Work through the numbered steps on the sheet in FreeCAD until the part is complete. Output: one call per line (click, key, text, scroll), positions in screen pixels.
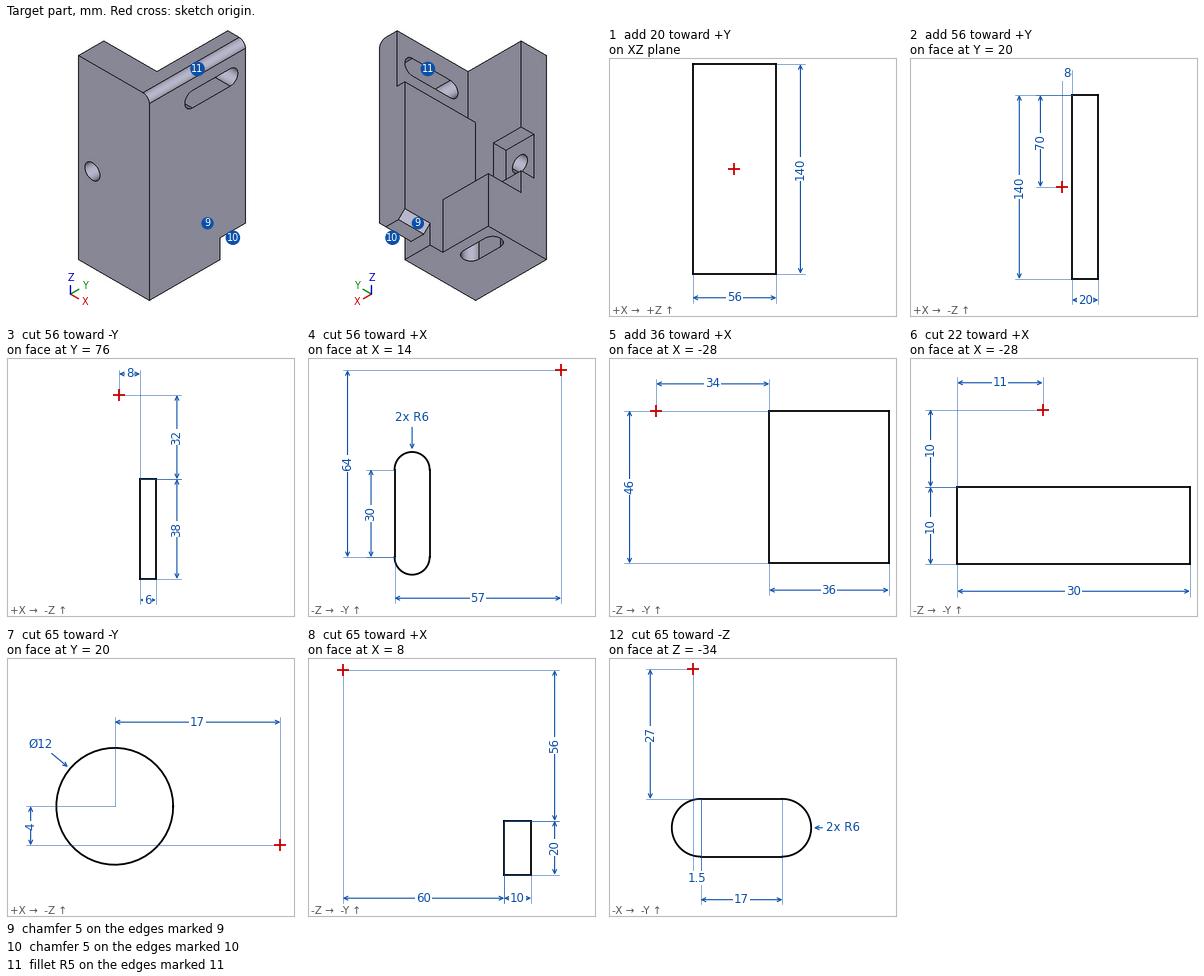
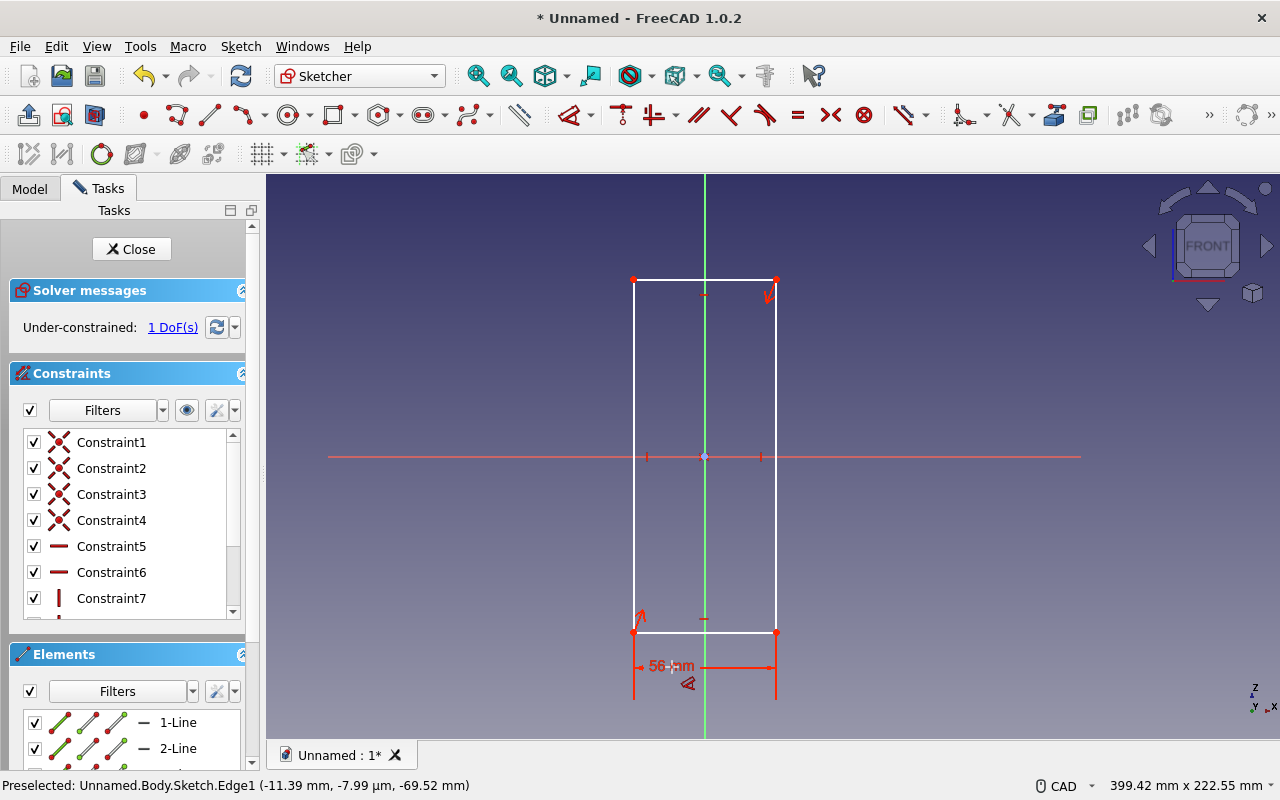
click(776, 527)
click(810, 375)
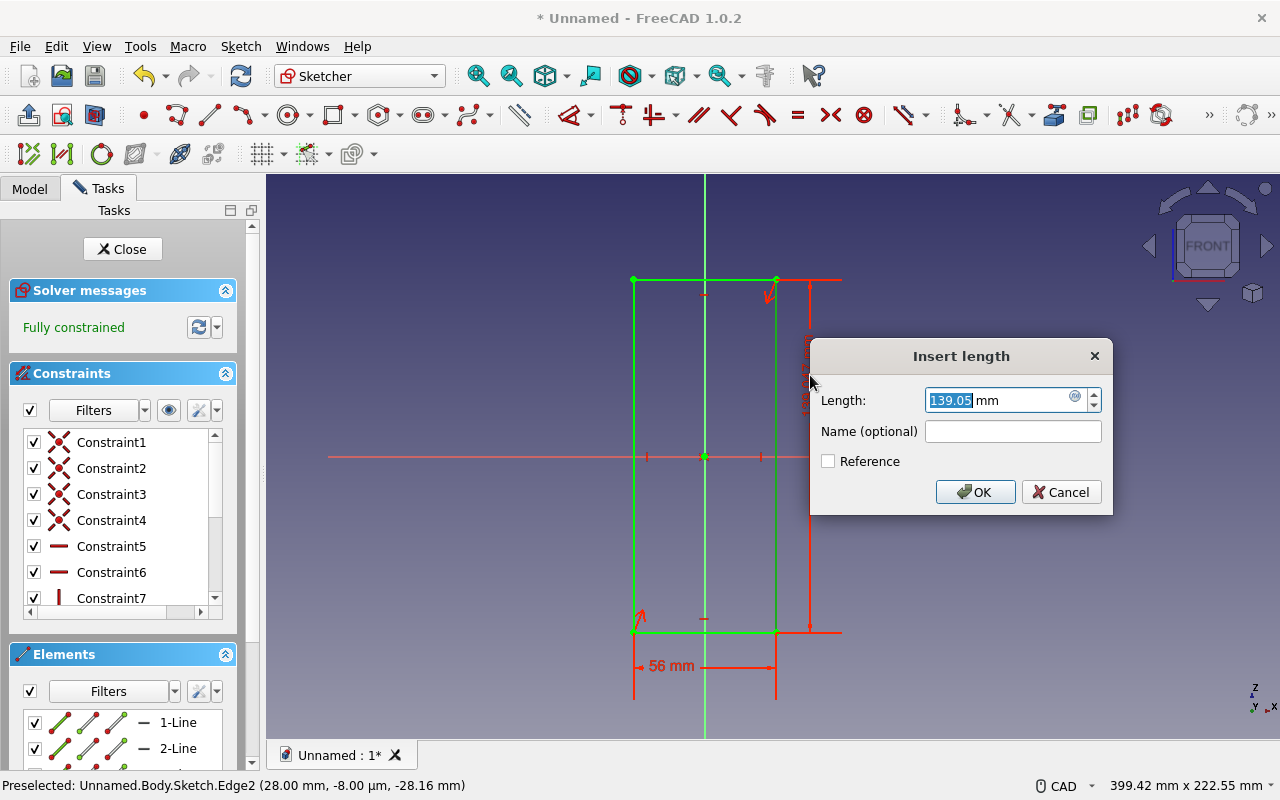
text(140)
key(Return)
key(Escape)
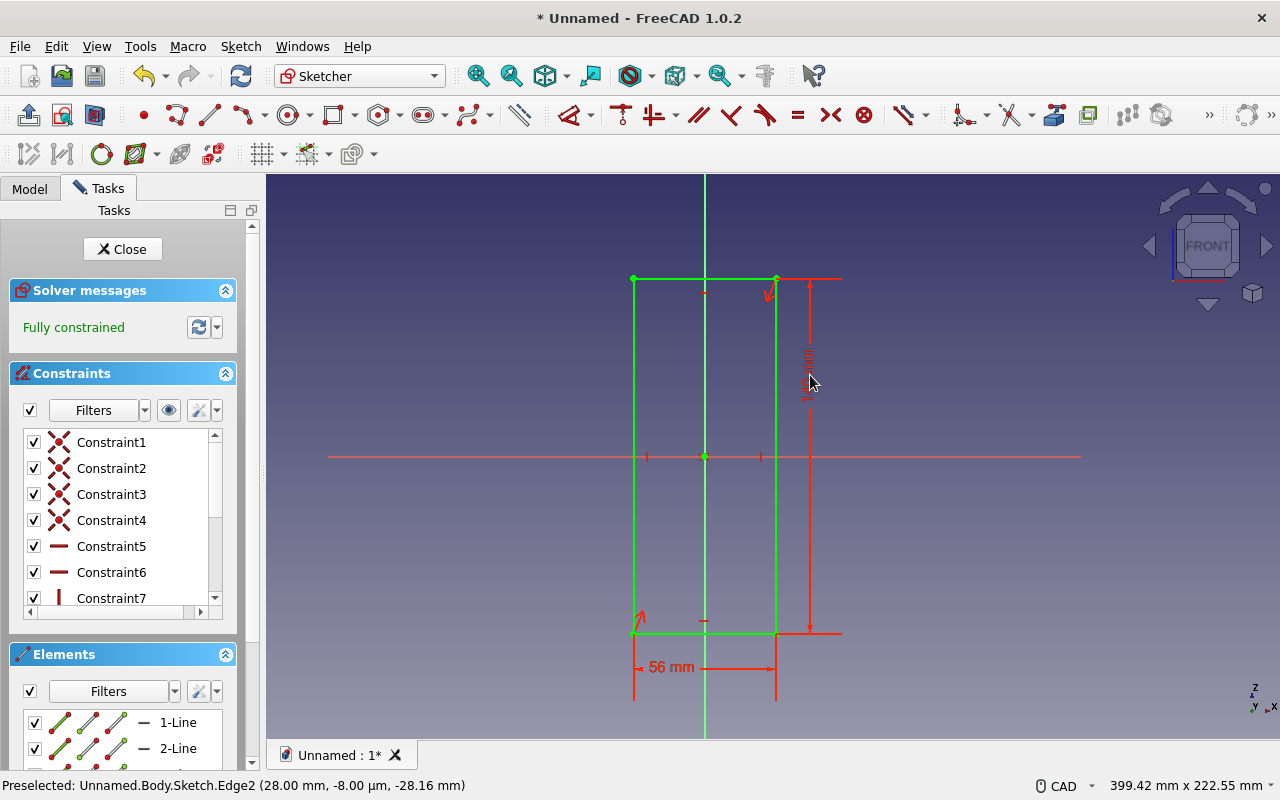
click(123, 249)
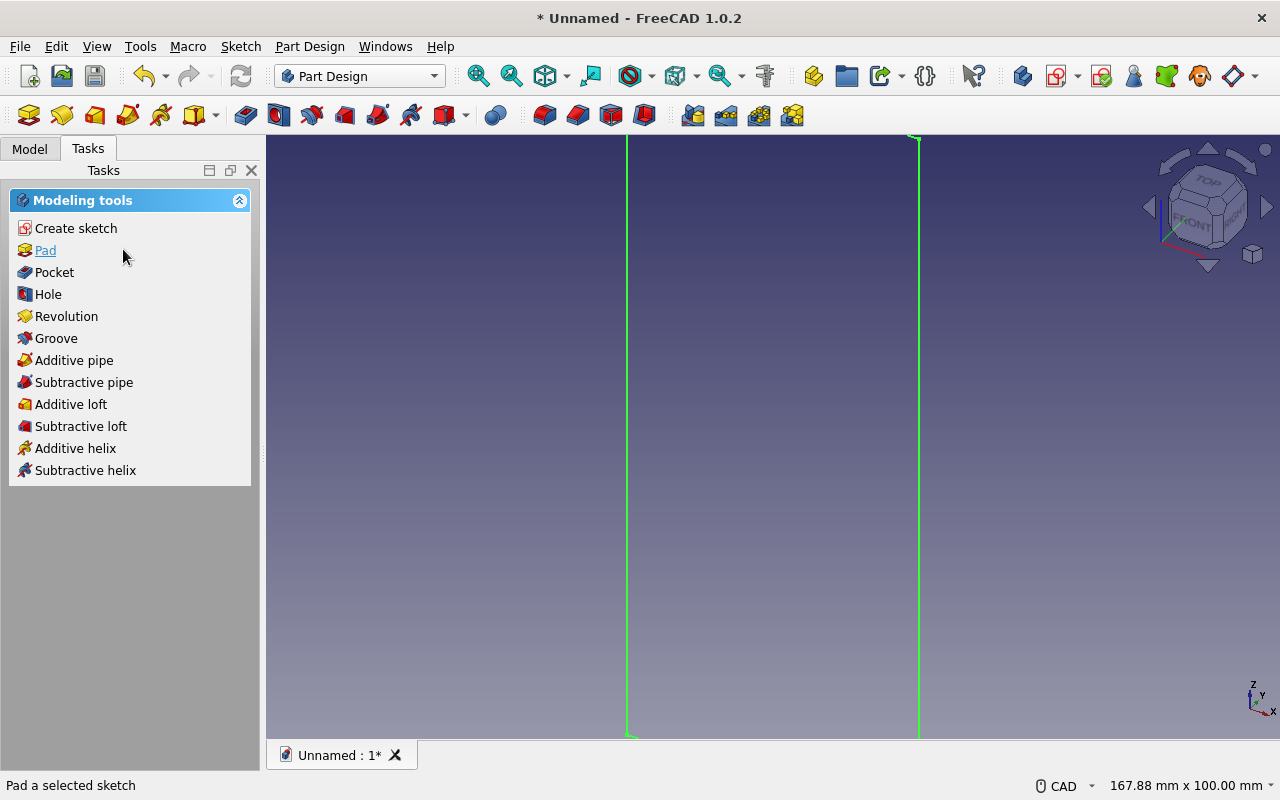
click(29, 116)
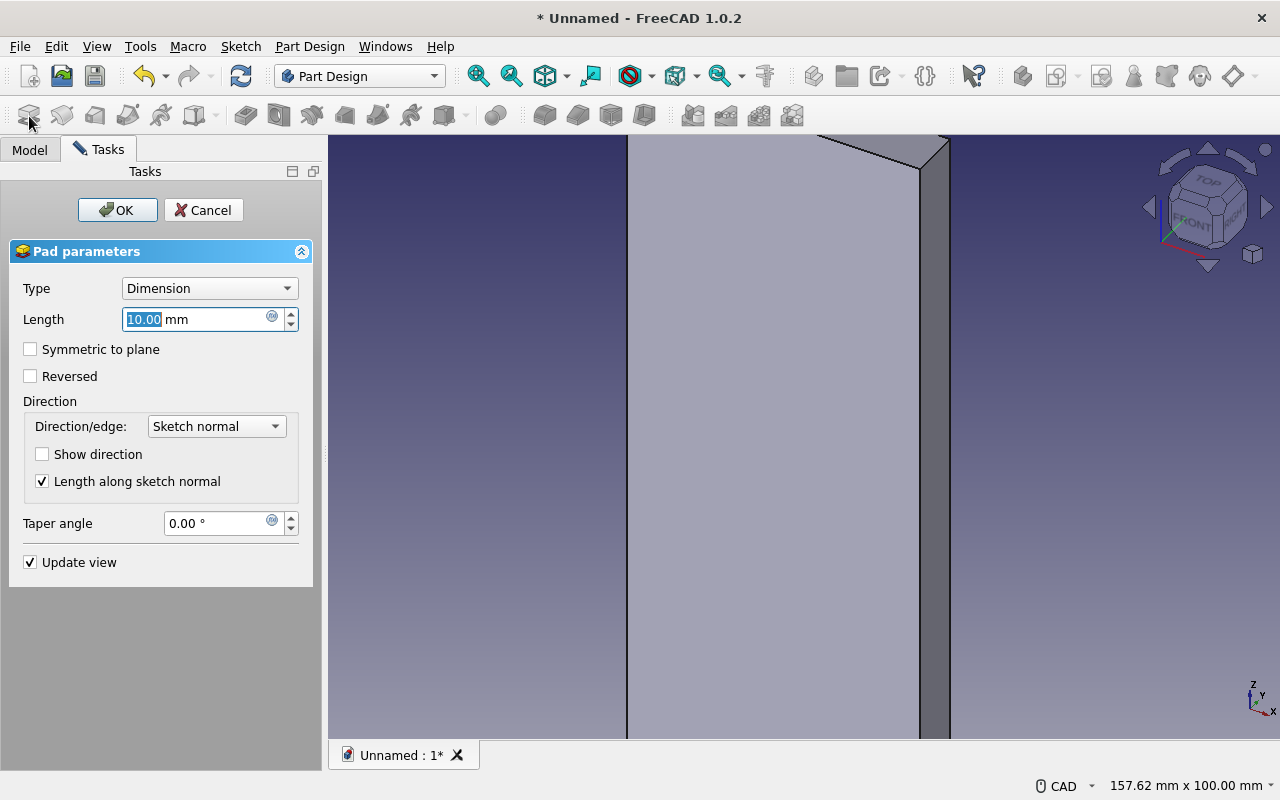
text(20)
key(Tab)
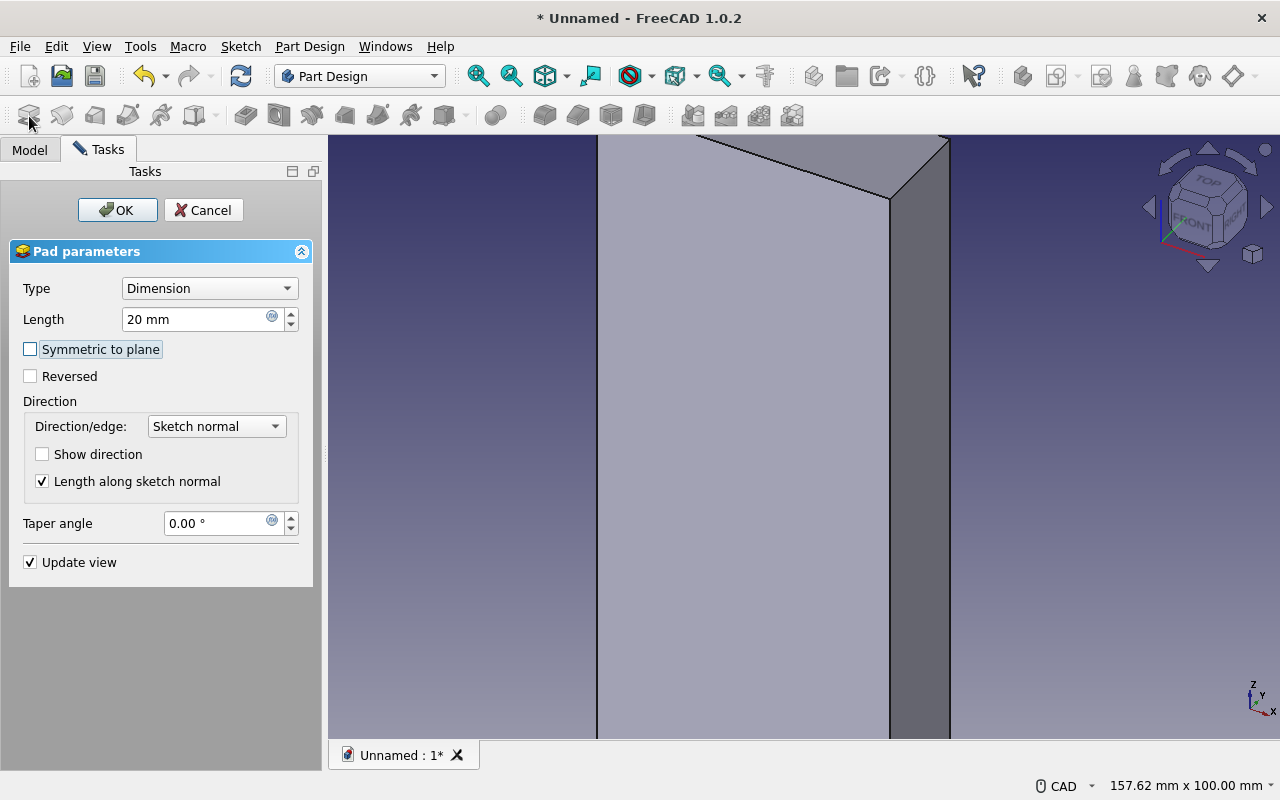
click(31, 376)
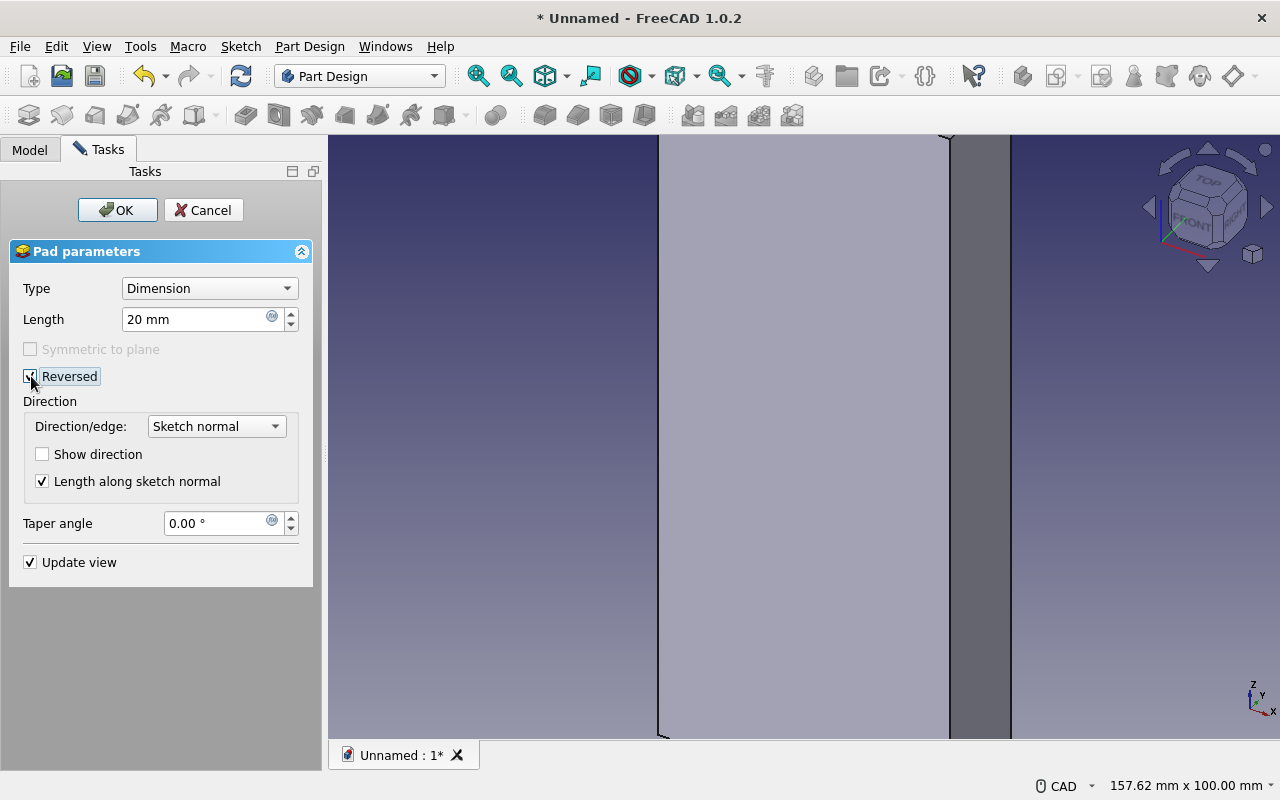
click(118, 210)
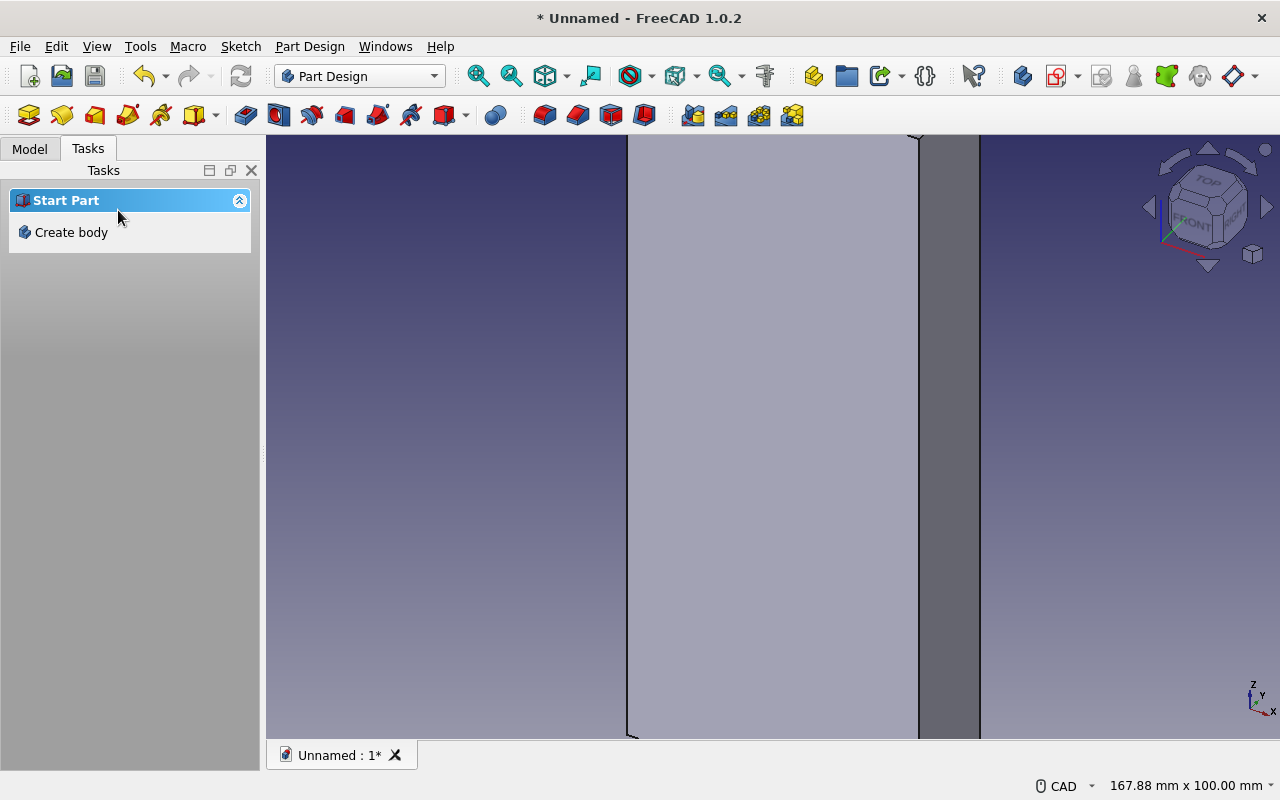
click(479, 76)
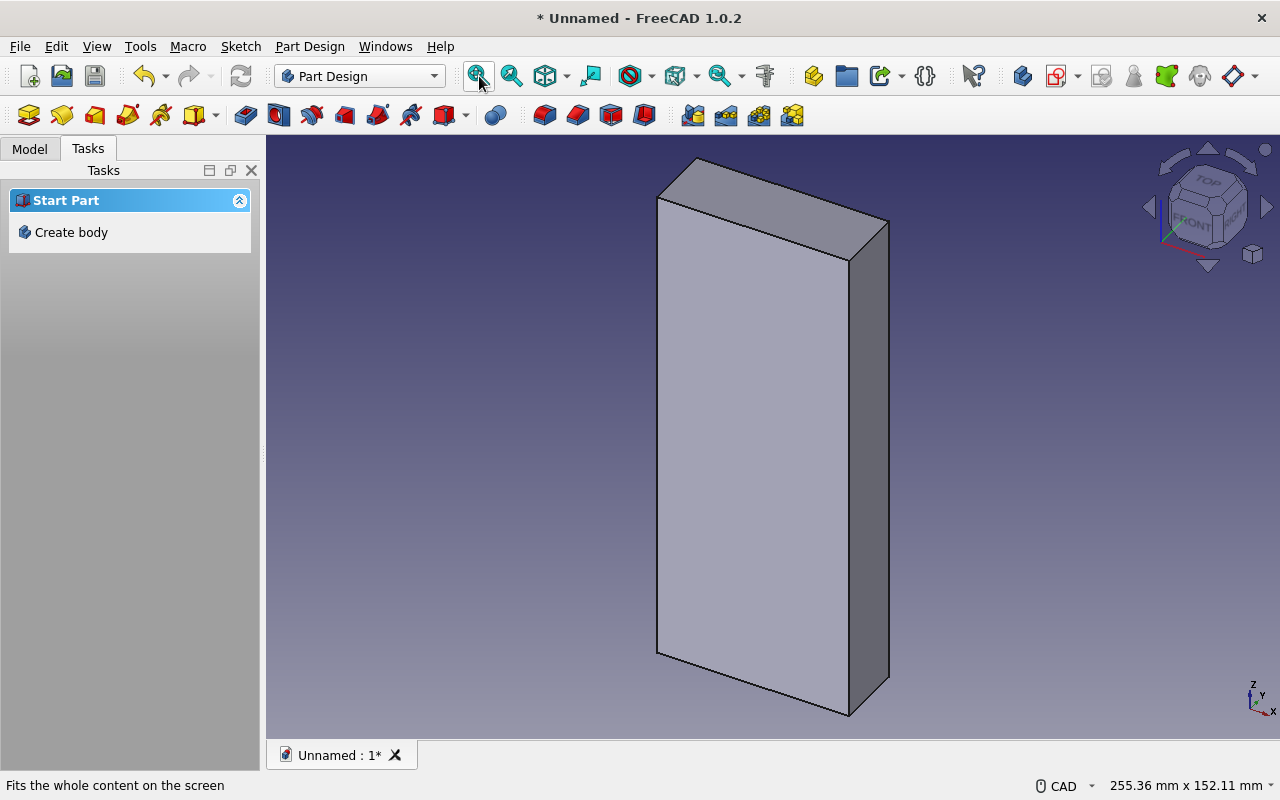
key(4)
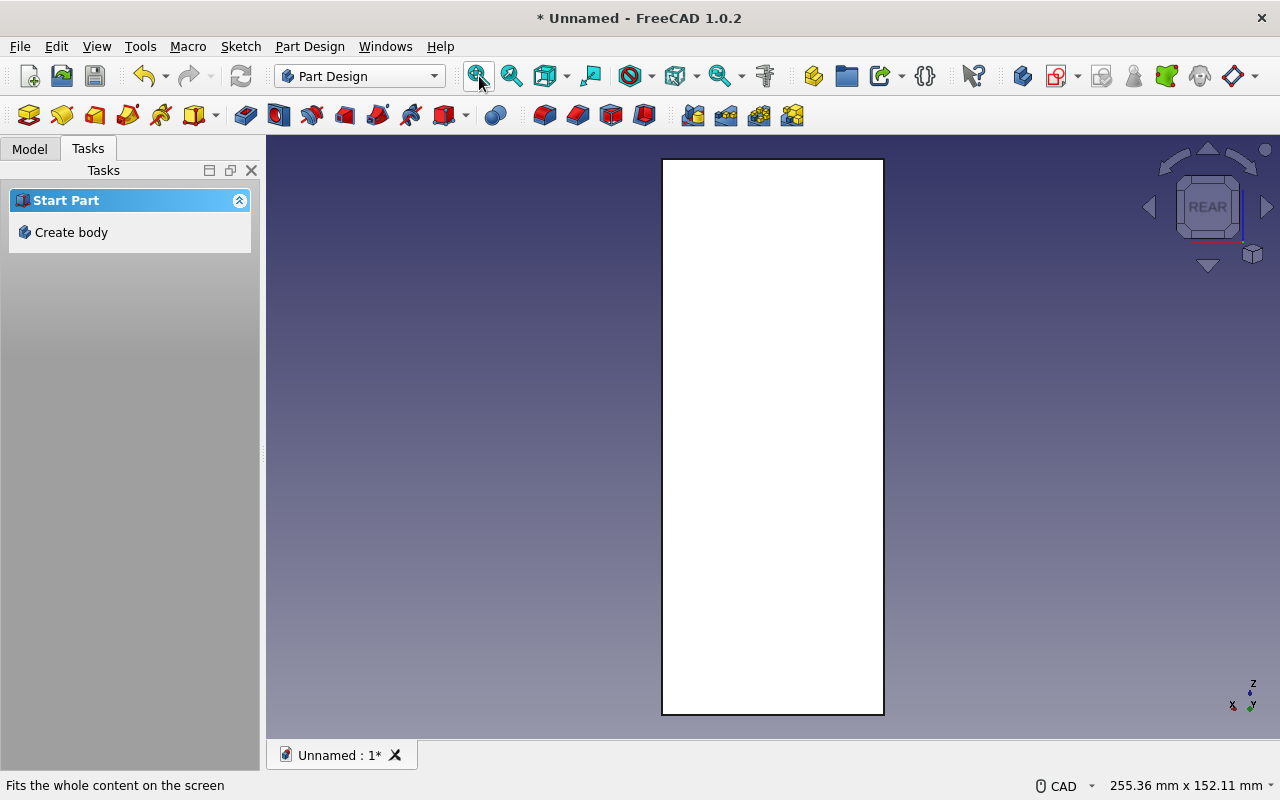
click(773, 277)